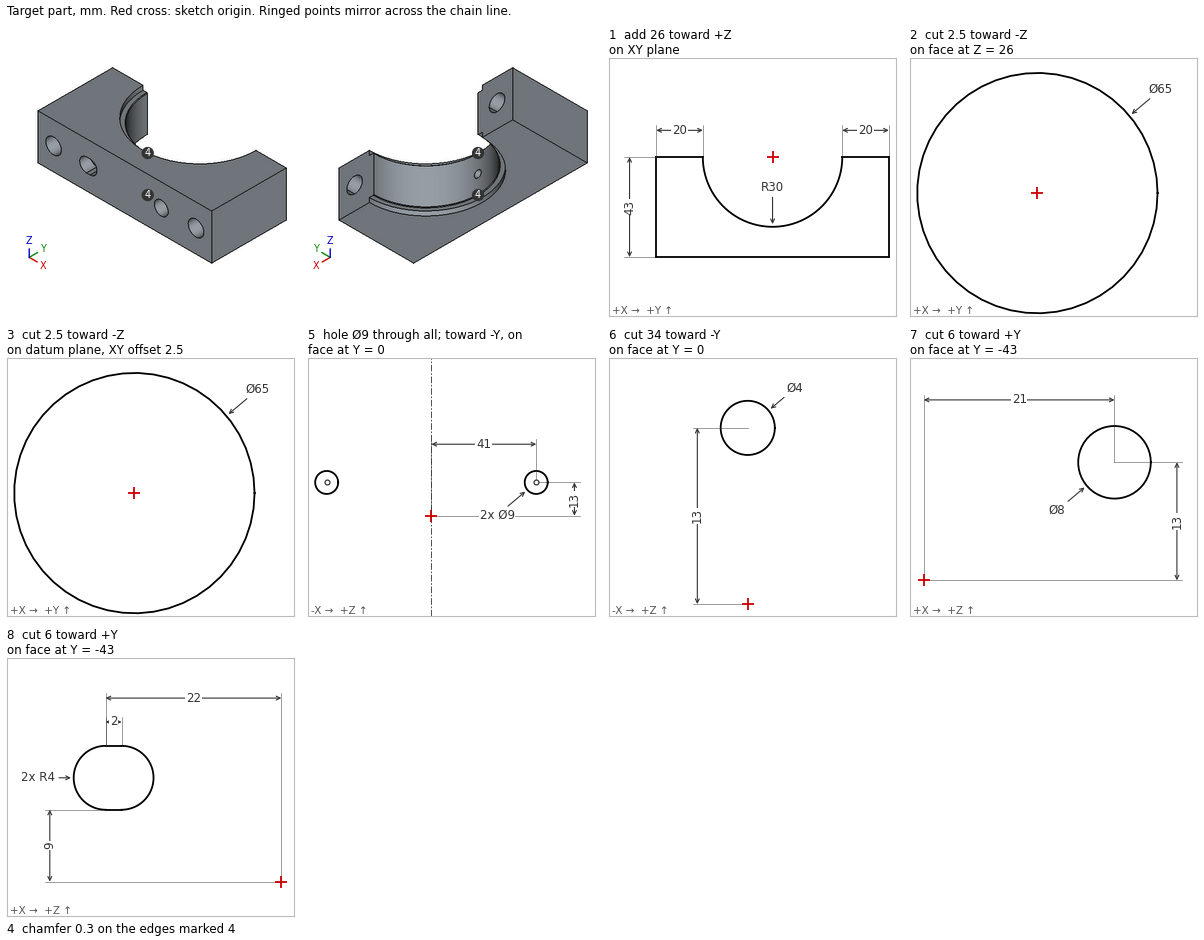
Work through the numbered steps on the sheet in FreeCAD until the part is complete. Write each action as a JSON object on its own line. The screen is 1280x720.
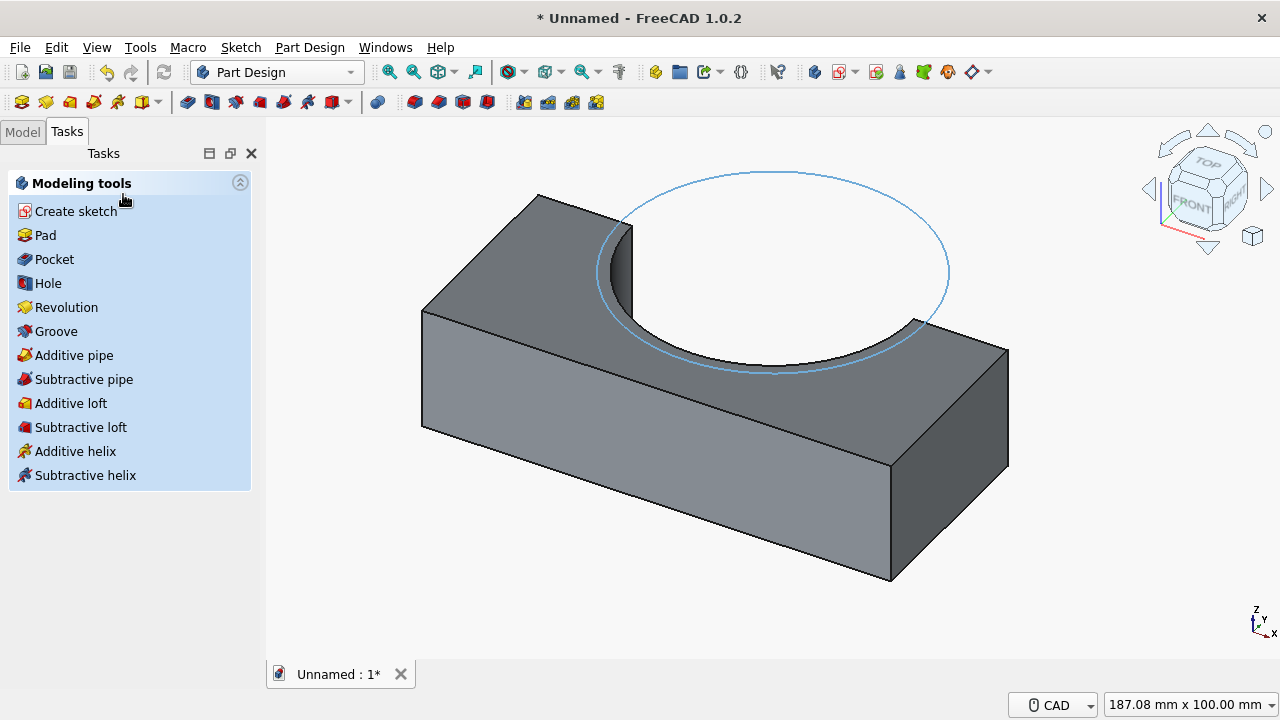
{"action": "left_click", "coordinate": [188, 102]}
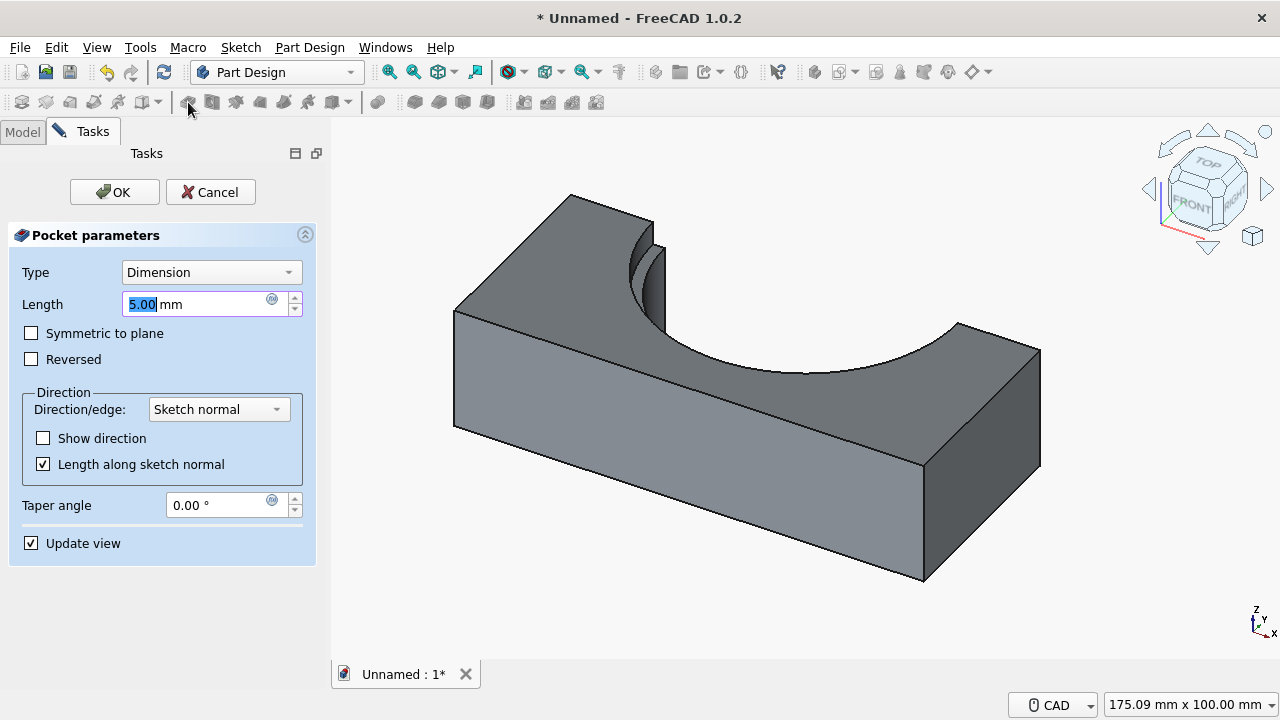
{"action": "type", "text": "2.5"}
{"action": "key", "text": "Tab"}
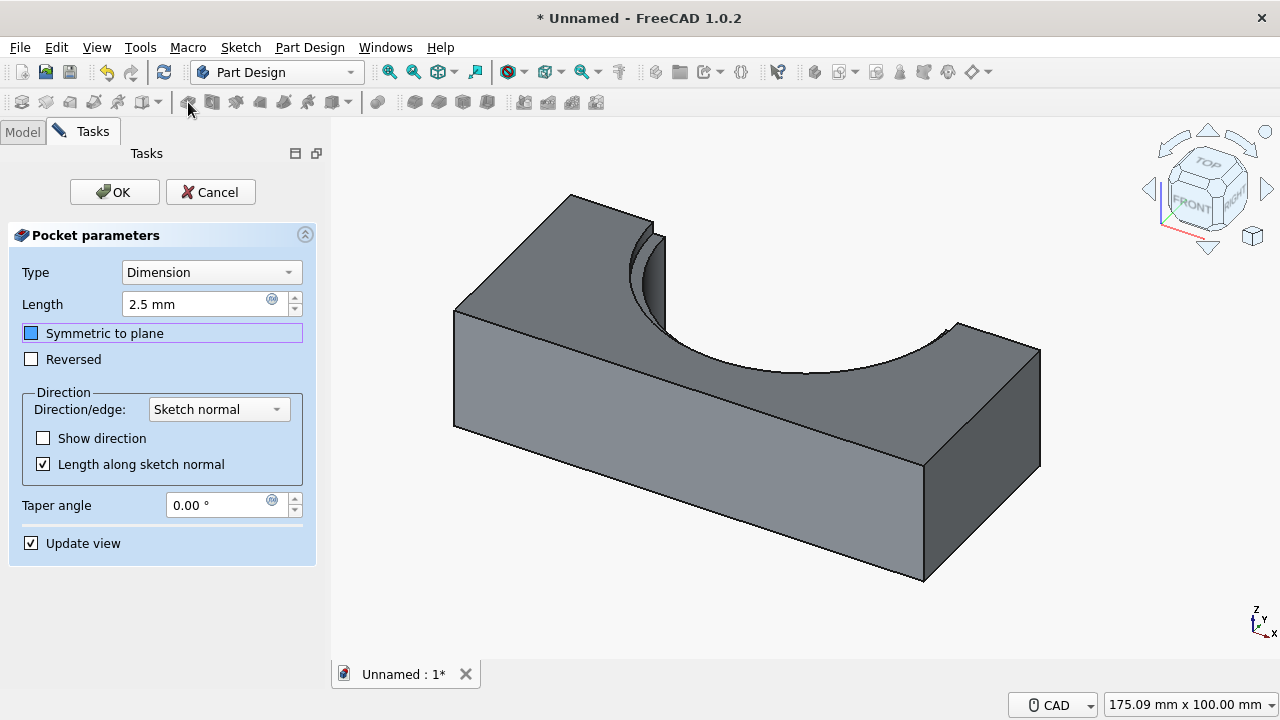
{"action": "left_click", "coordinate": [115, 192]}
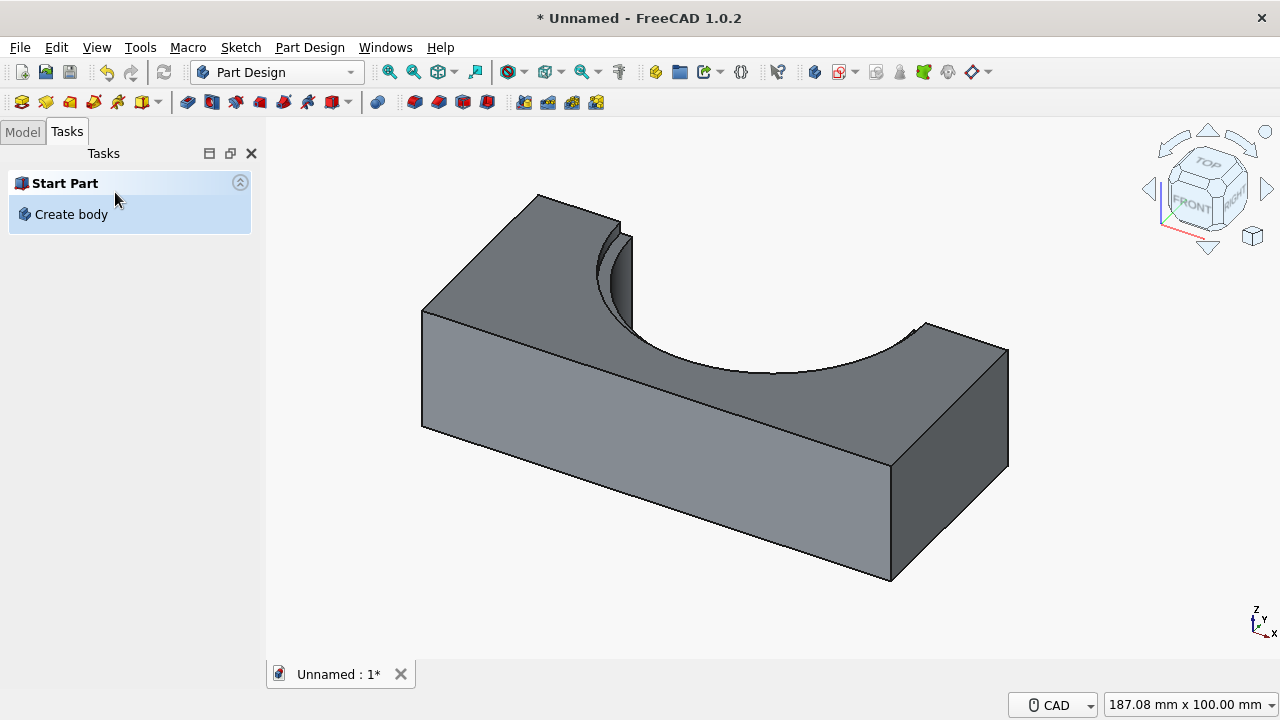
{"action": "left_click", "coordinate": [23, 131]}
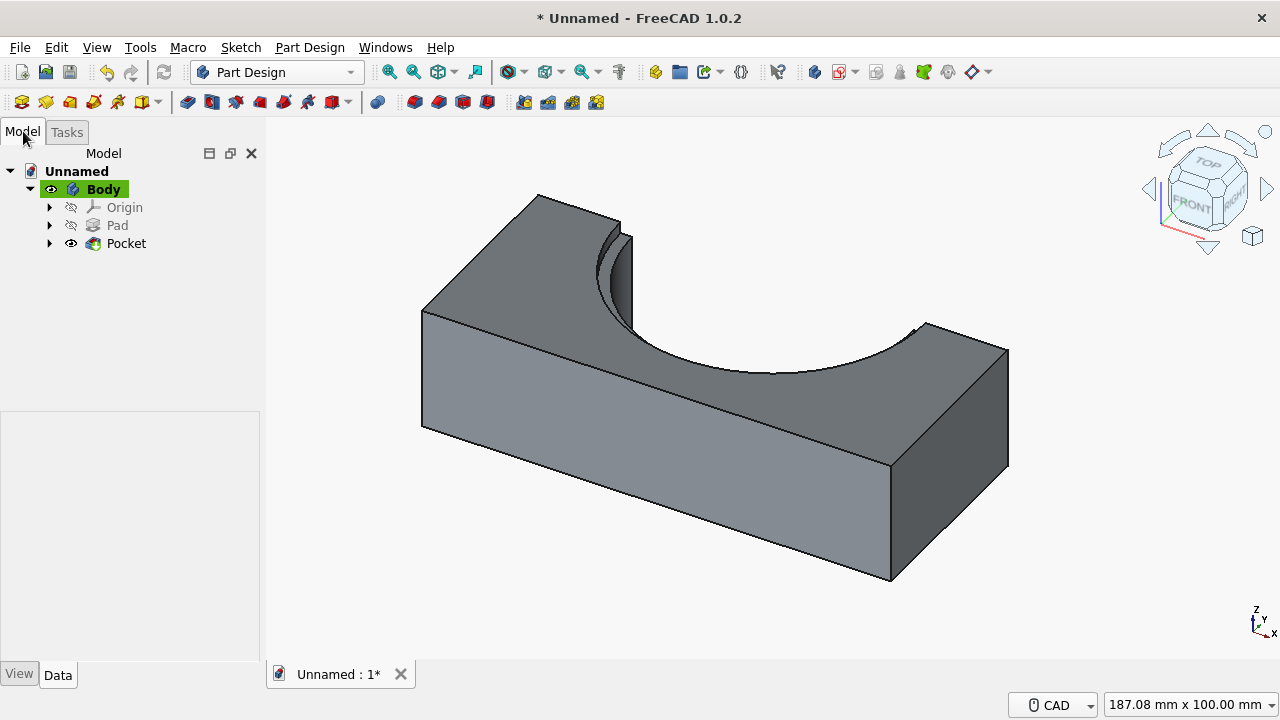
{"action": "left_click", "coordinate": [50, 207]}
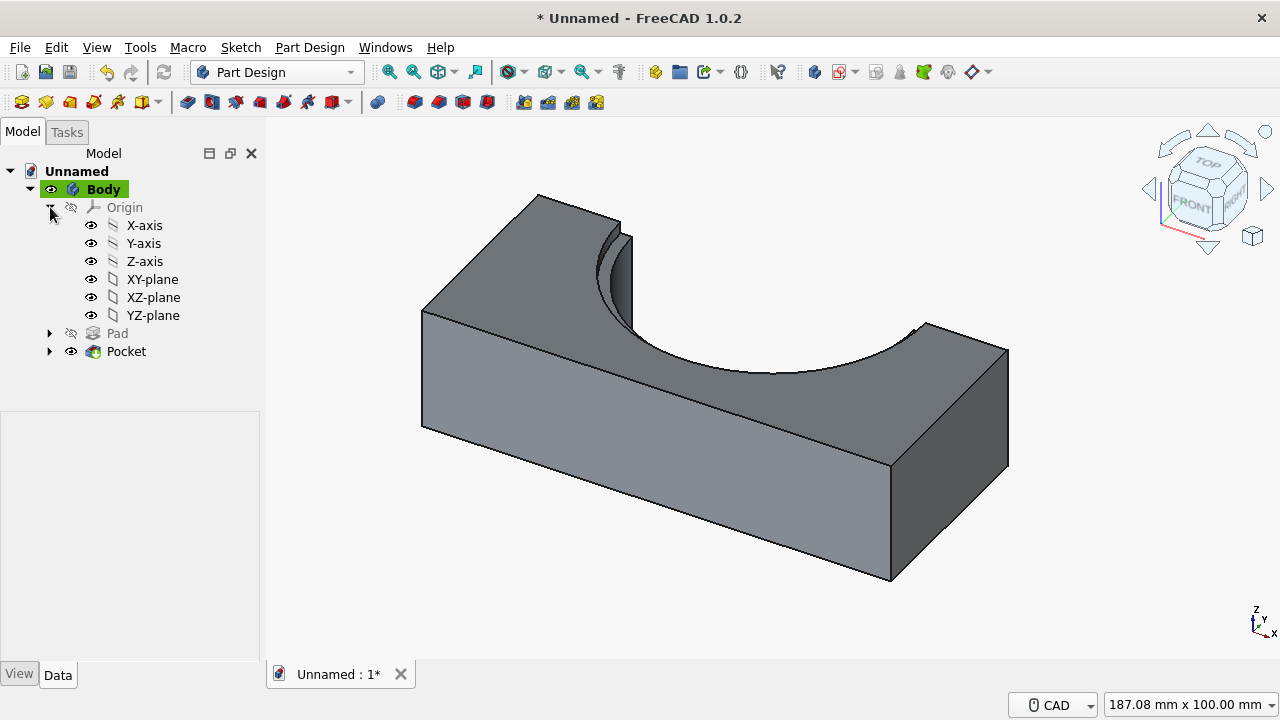
{"action": "left_click", "coordinate": [136, 279]}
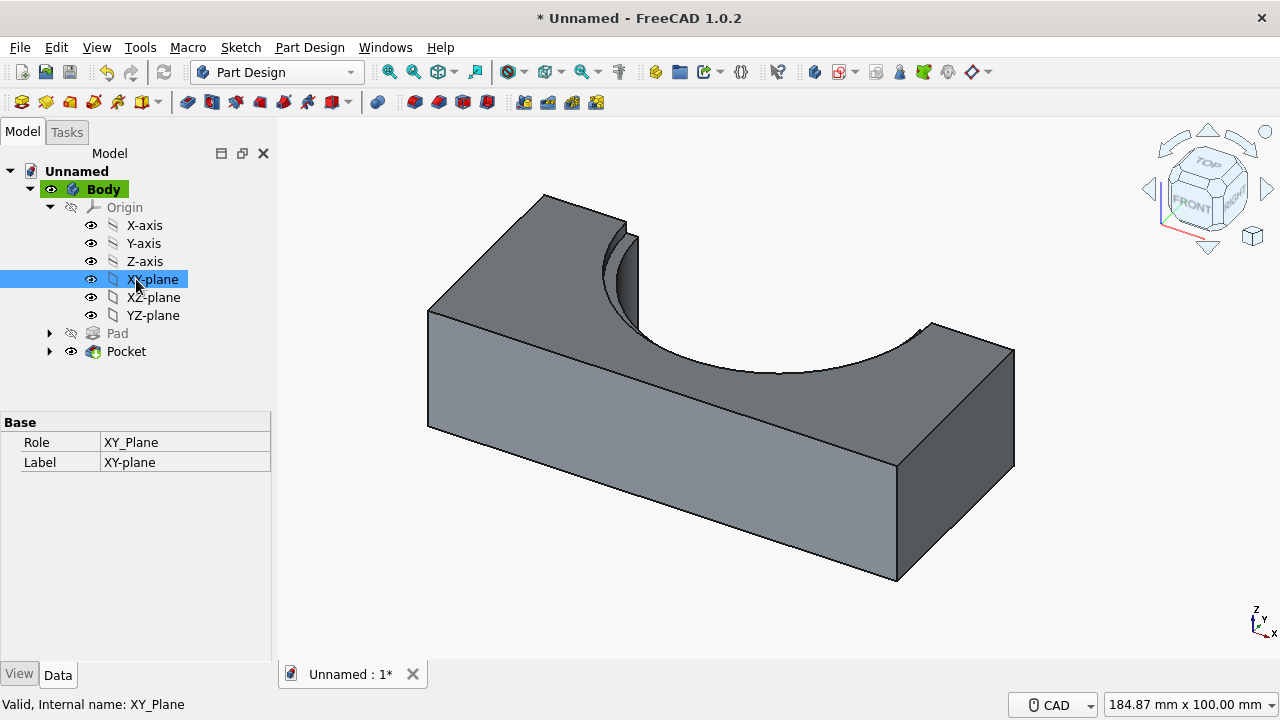
{"action": "left_click", "coordinate": [972, 72]}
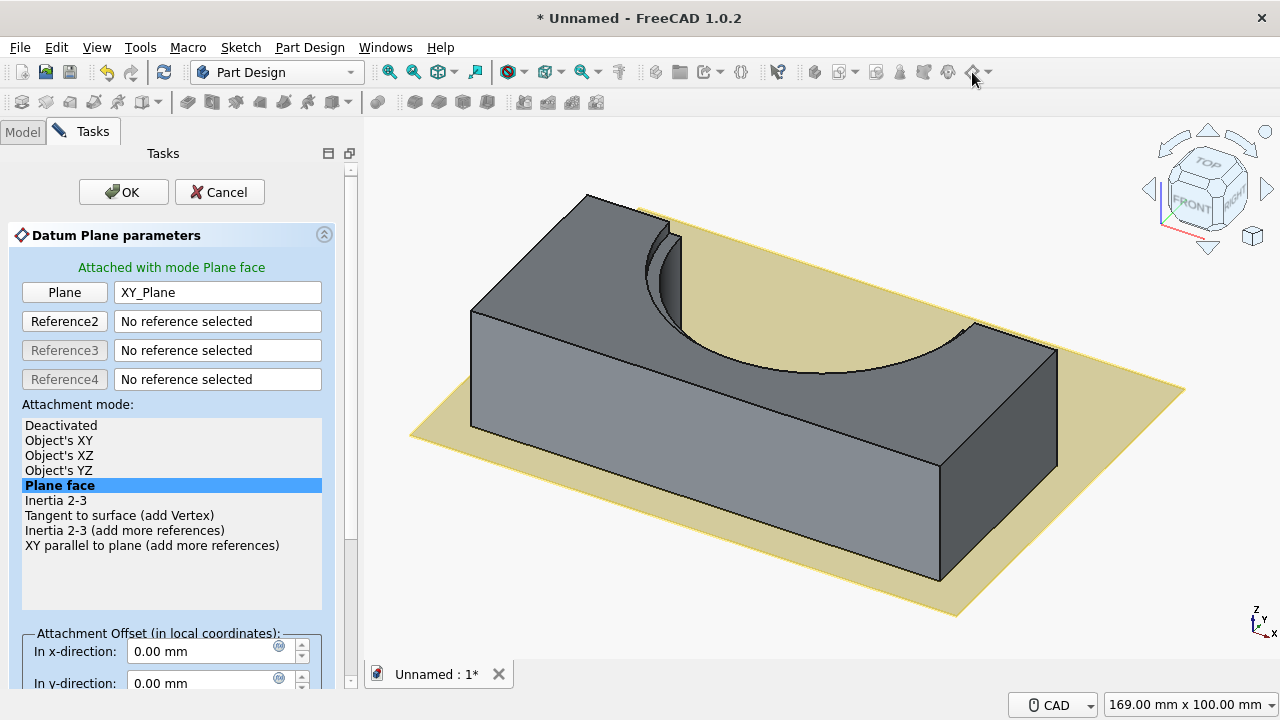
{"action": "scroll", "coordinate": [351, 426], "scroll_direction": "down", "scroll_amount": 2}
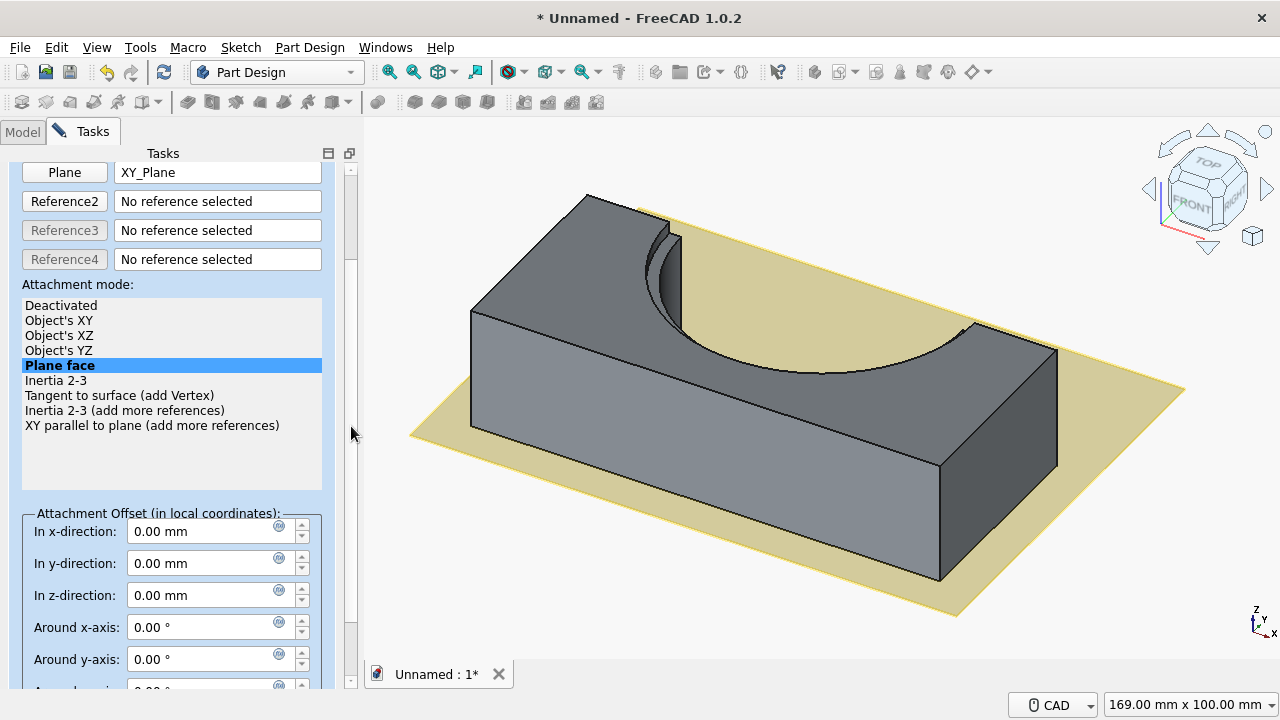
{"action": "triple_click", "coordinate": [210, 595]}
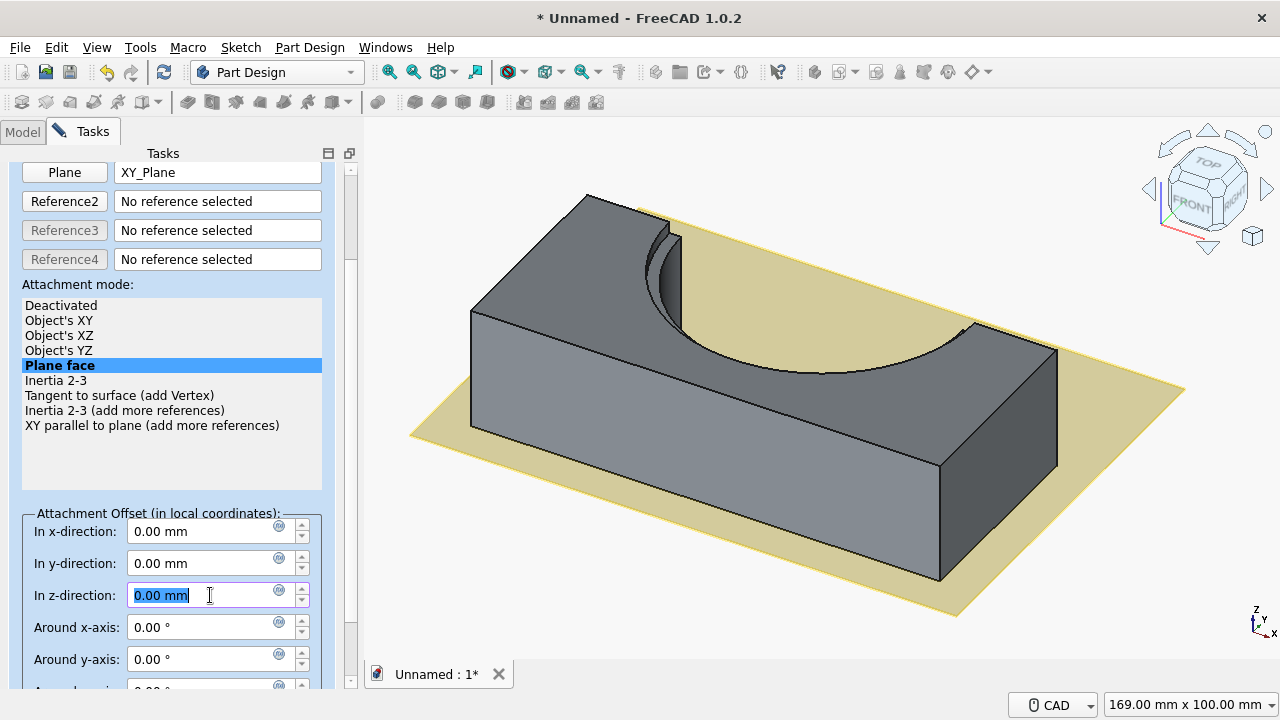
{"action": "type", "text": "2.5"}
{"action": "key", "text": "Tab"}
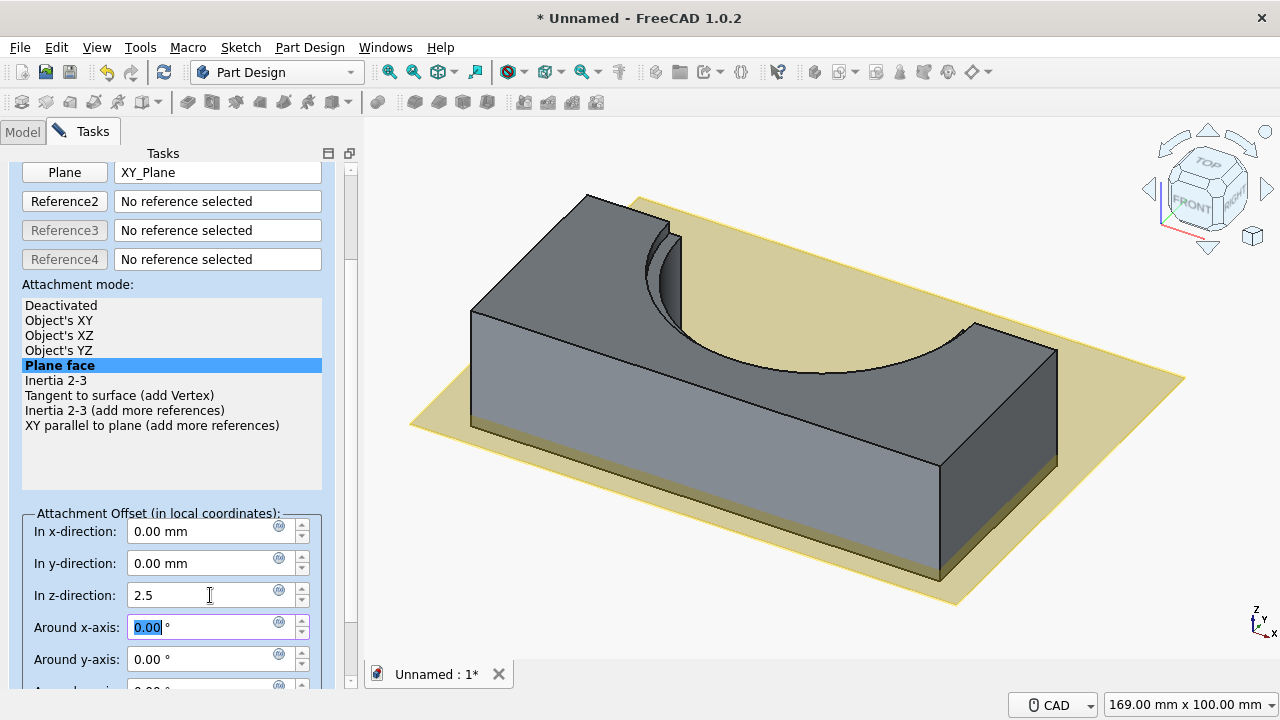
{"action": "scroll", "coordinate": [351, 426], "scroll_direction": "up", "scroll_amount": 3}